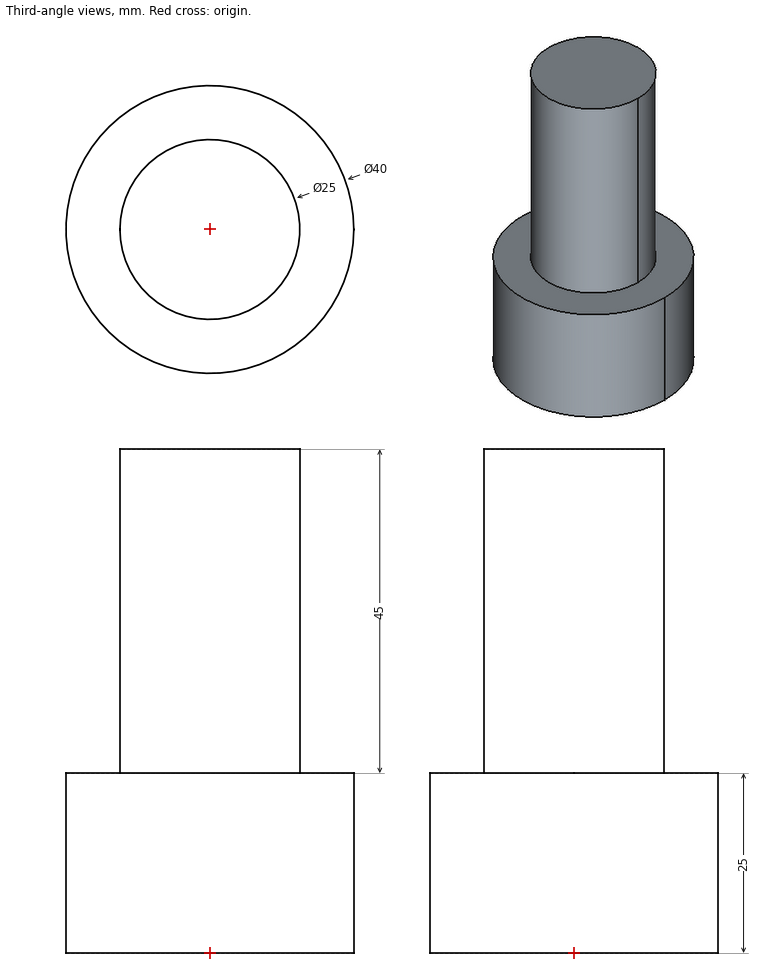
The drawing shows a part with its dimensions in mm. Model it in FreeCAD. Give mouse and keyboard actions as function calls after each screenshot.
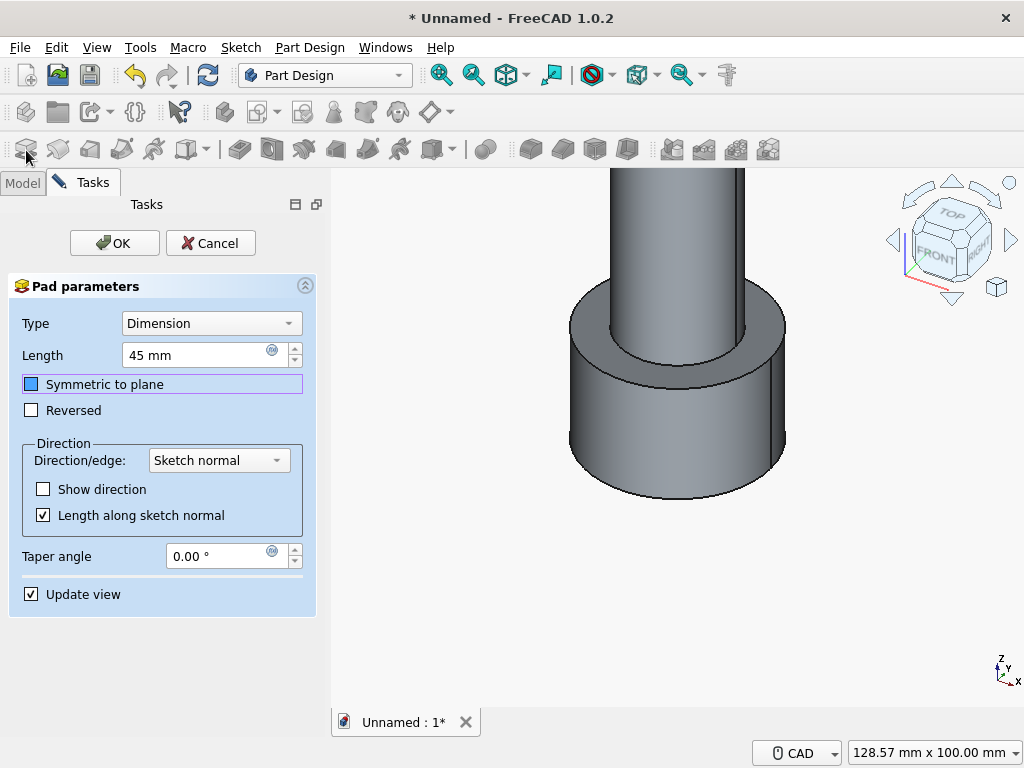
click(115, 243)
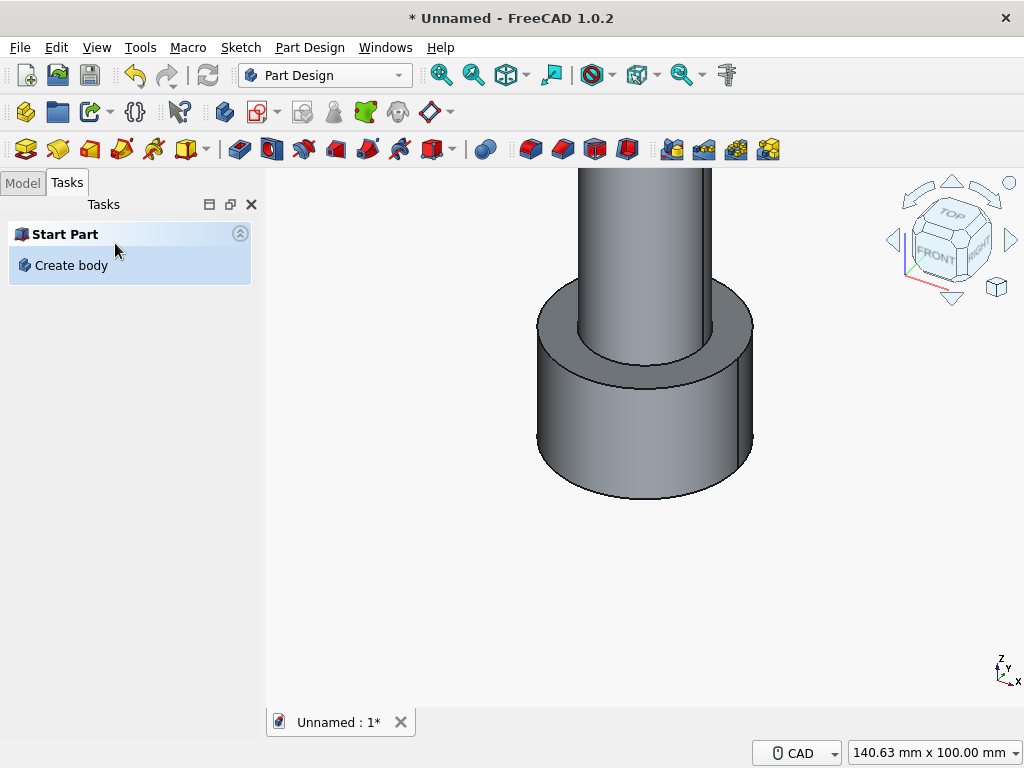
key(0)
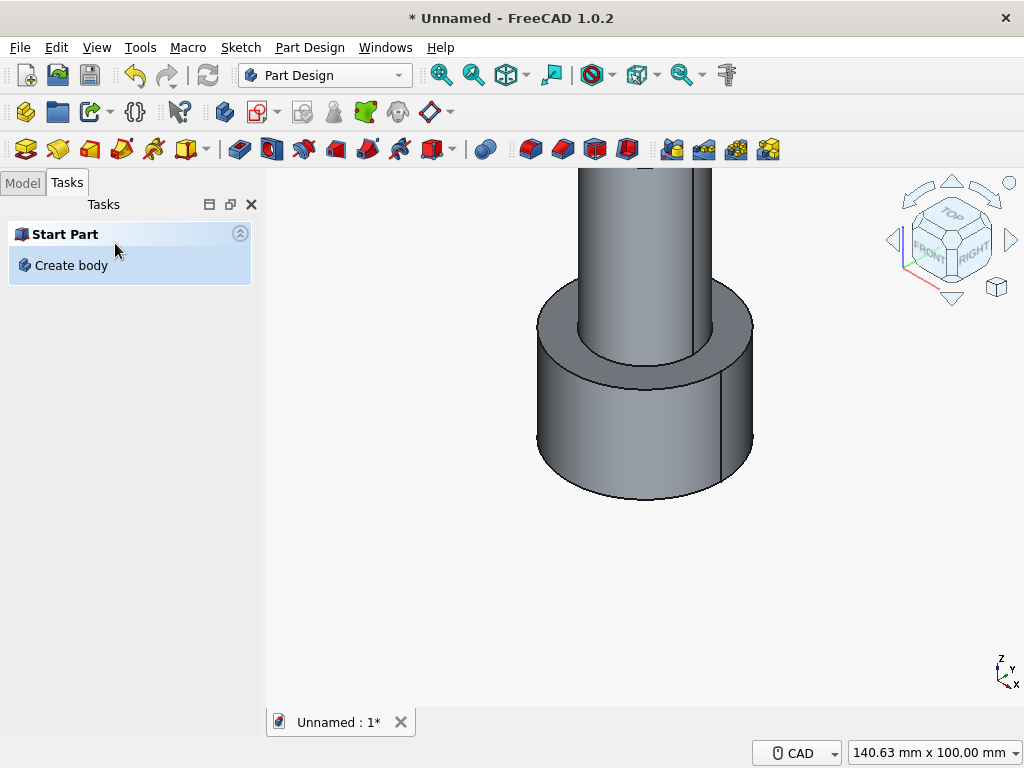
click(442, 76)